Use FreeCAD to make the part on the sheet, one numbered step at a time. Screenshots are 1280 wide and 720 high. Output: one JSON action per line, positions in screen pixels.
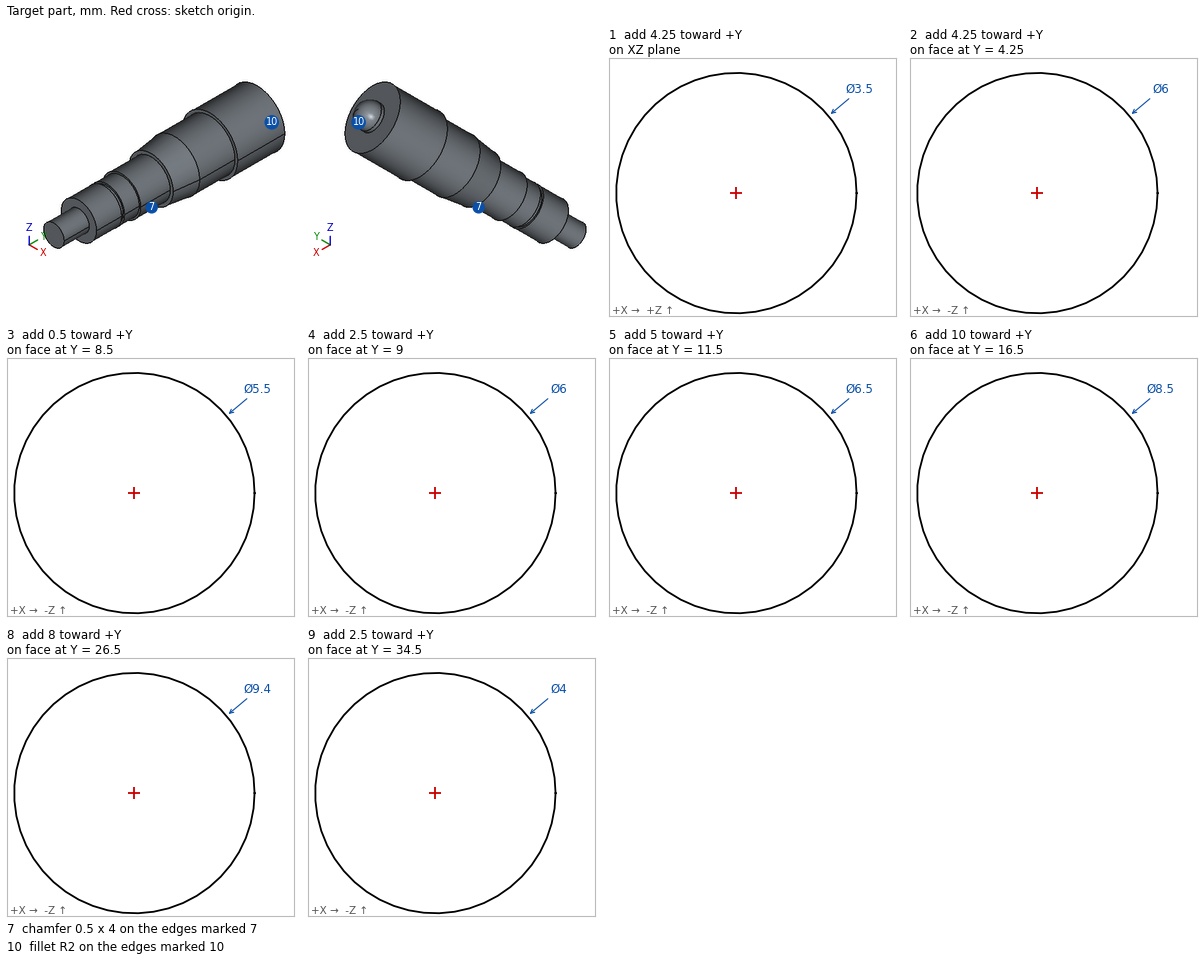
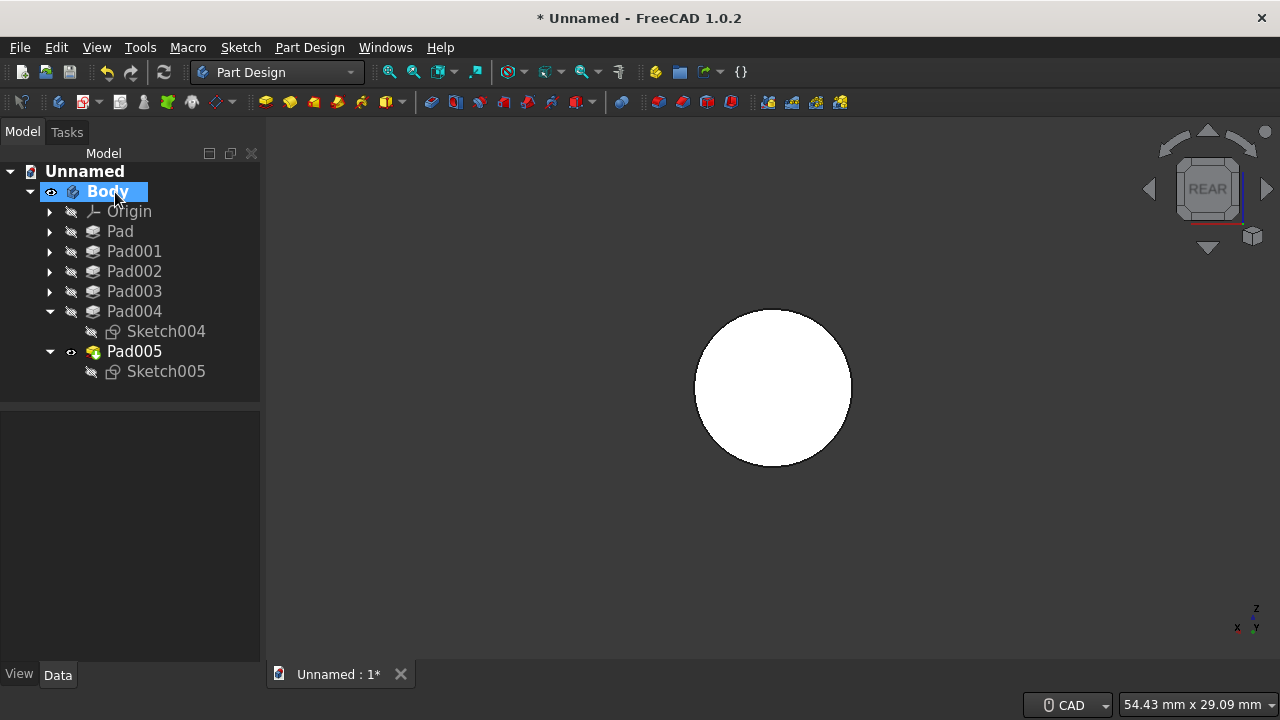
{"action": "key", "text": "0"}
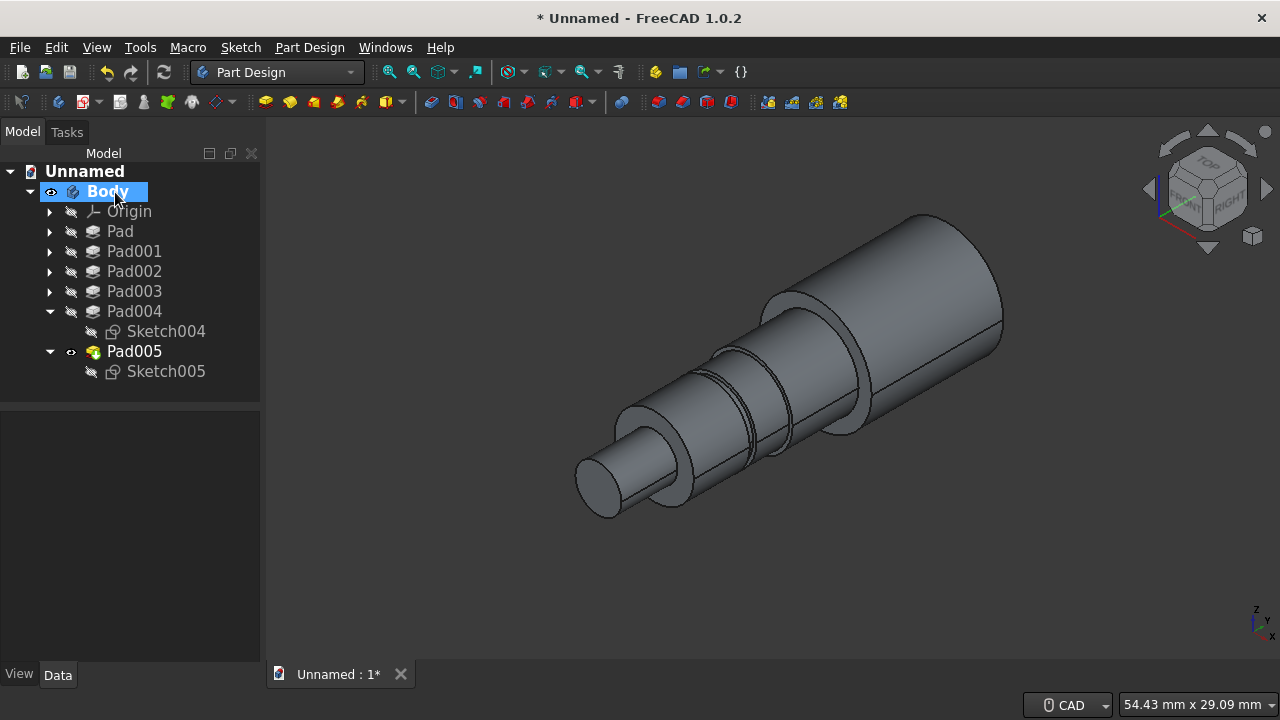
{"action": "left_click", "coordinate": [798, 291]}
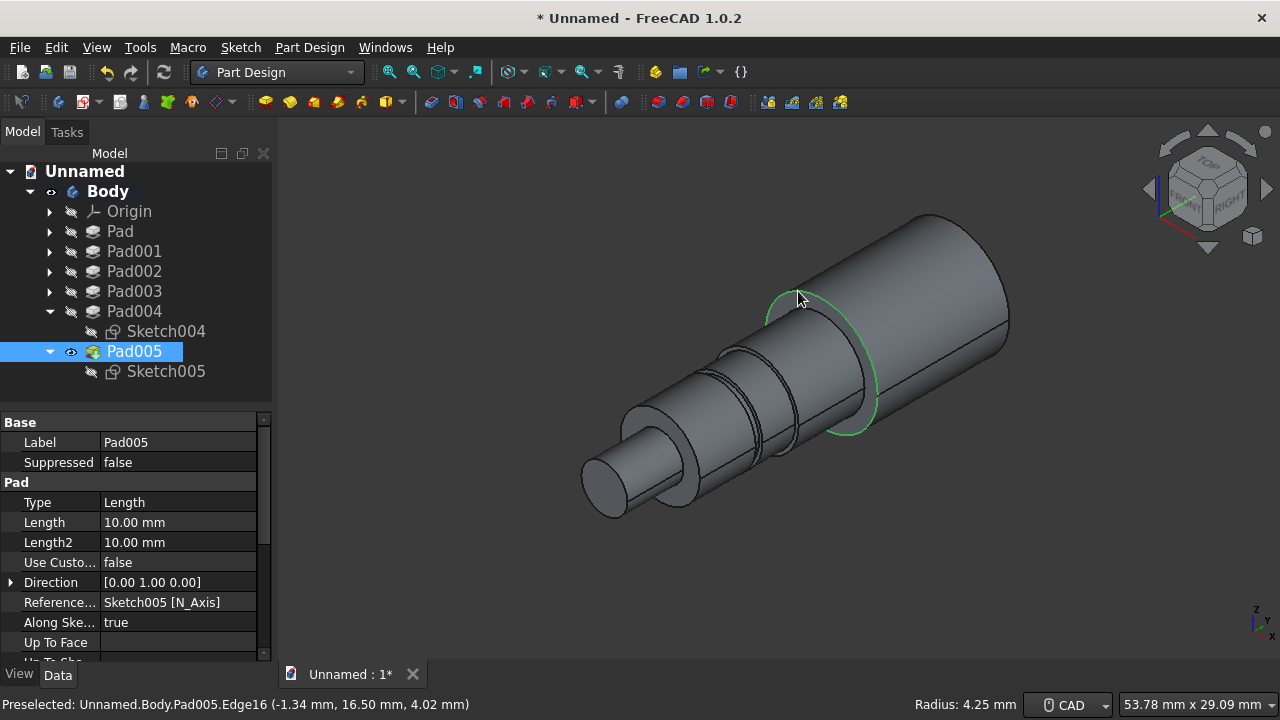
{"action": "left_click", "coordinate": [684, 102]}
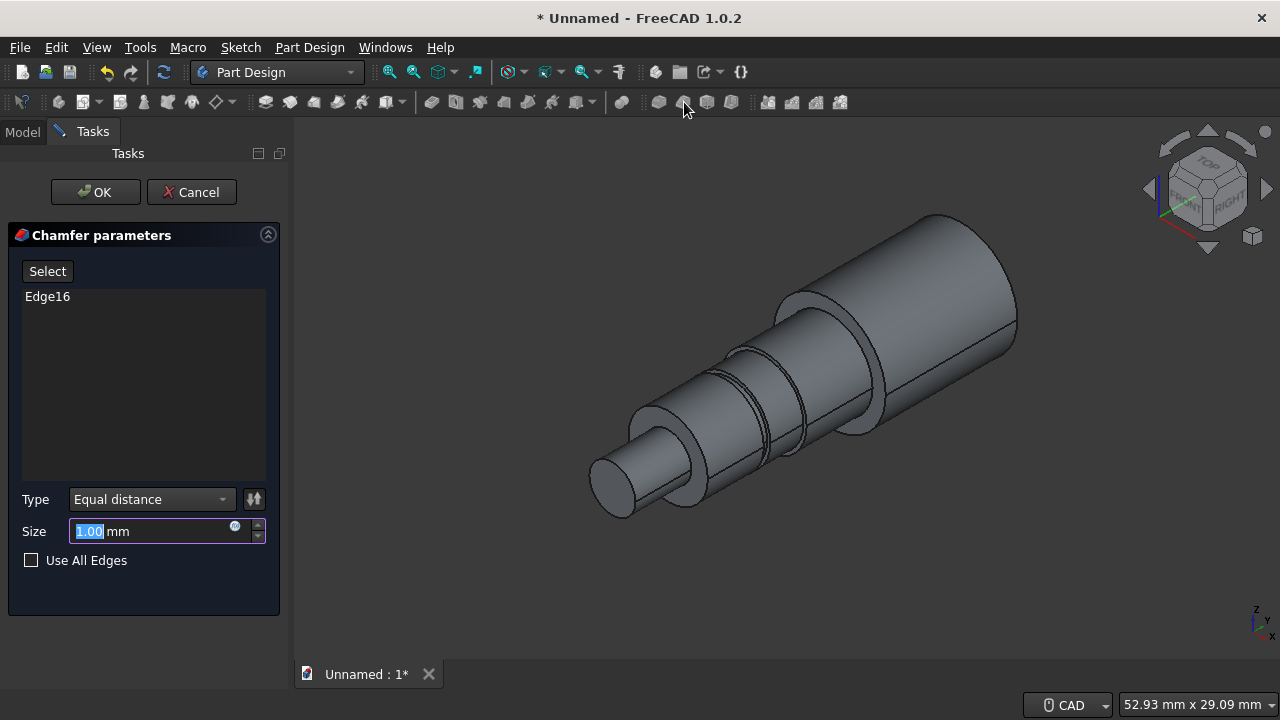
{"action": "type", "text": "0.5"}
{"action": "key", "text": "Tab"}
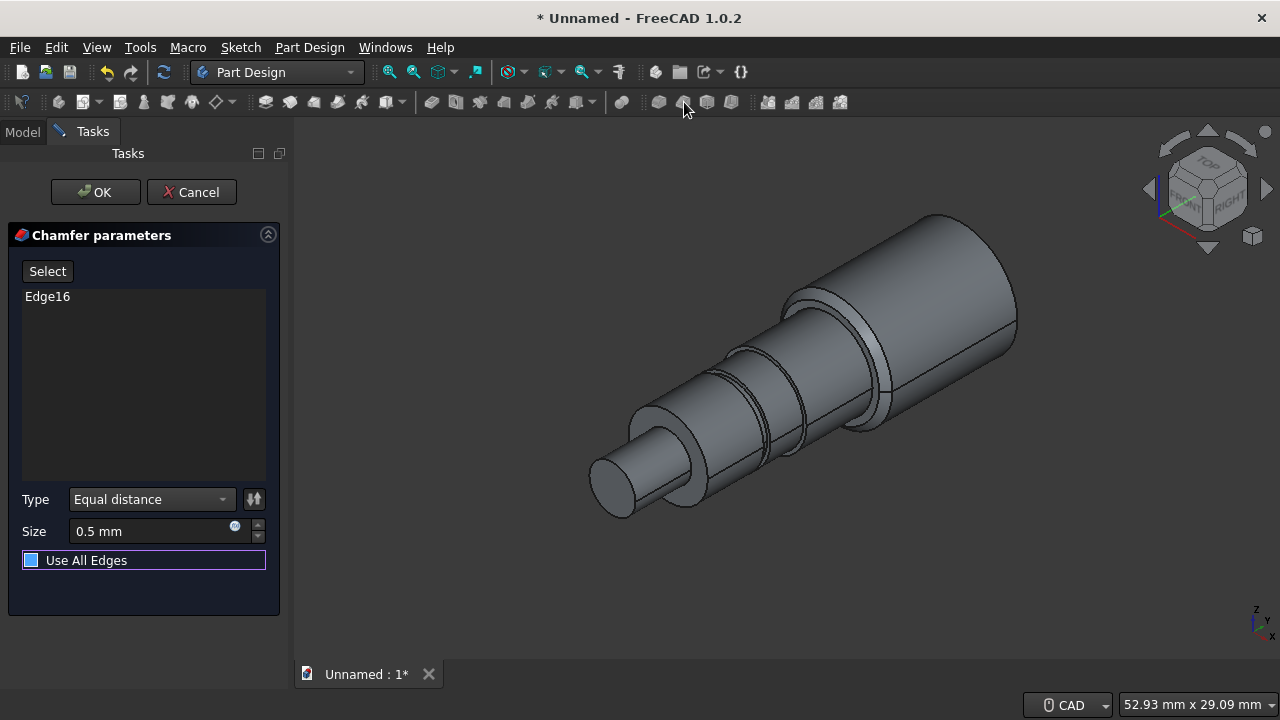
{"action": "left_click", "coordinate": [153, 500]}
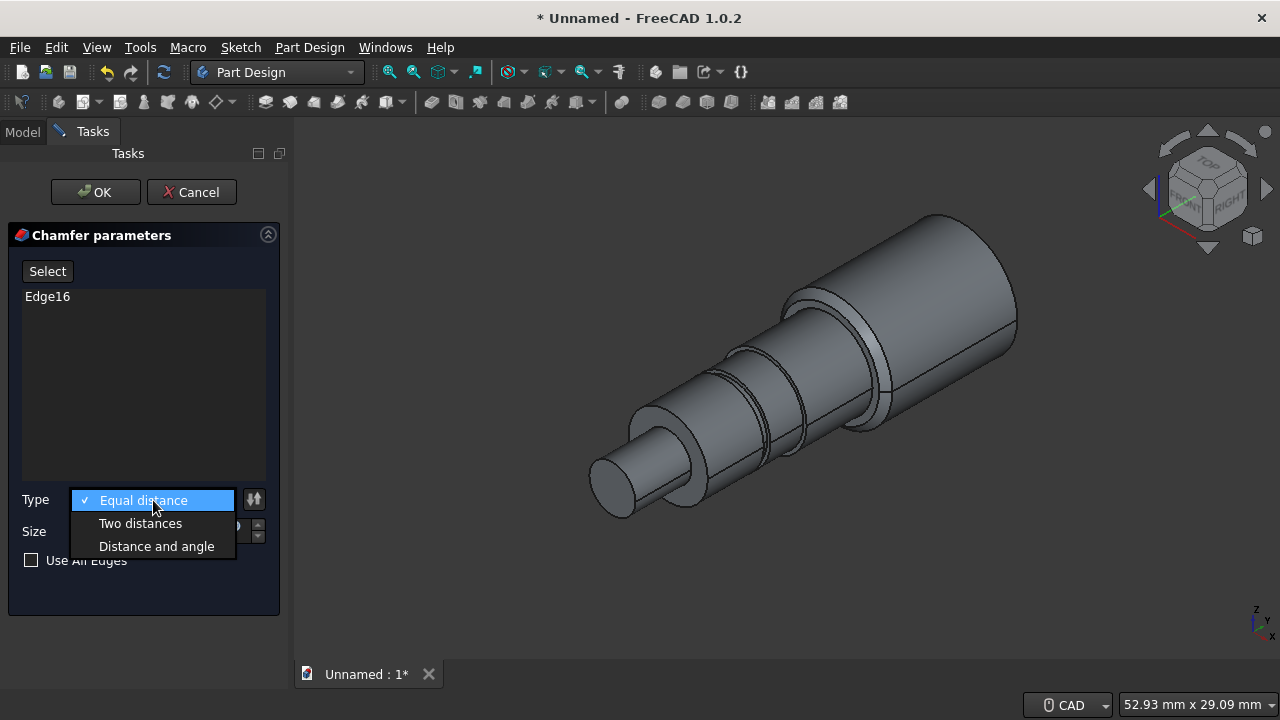
{"action": "left_click", "coordinate": [152, 524]}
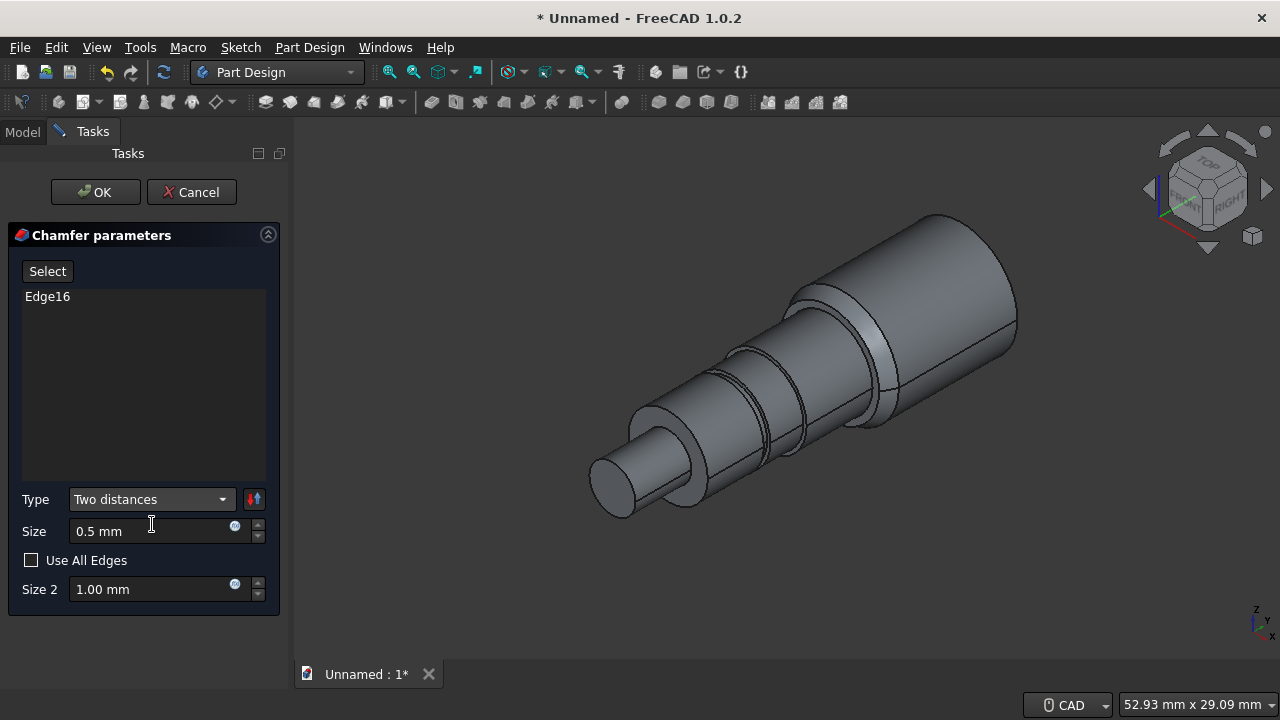
{"action": "triple_click", "coordinate": [160, 589]}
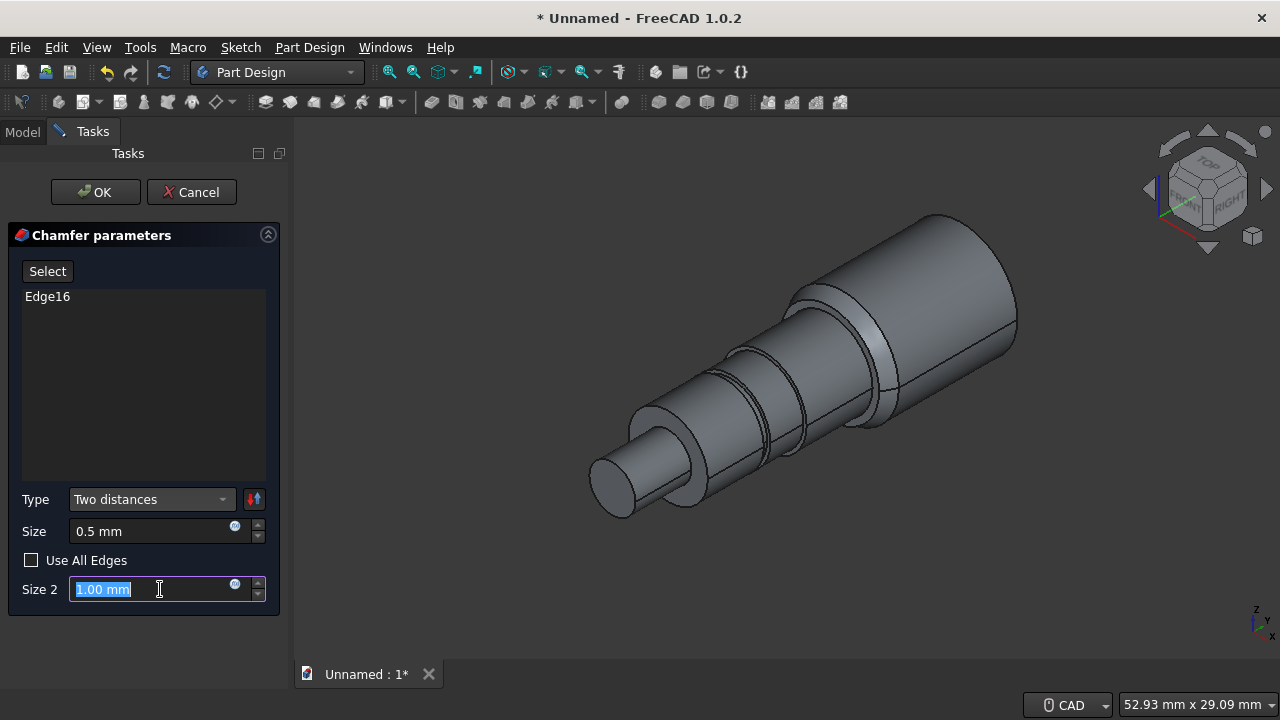
{"action": "type", "text": "4"}
{"action": "key", "text": "Tab"}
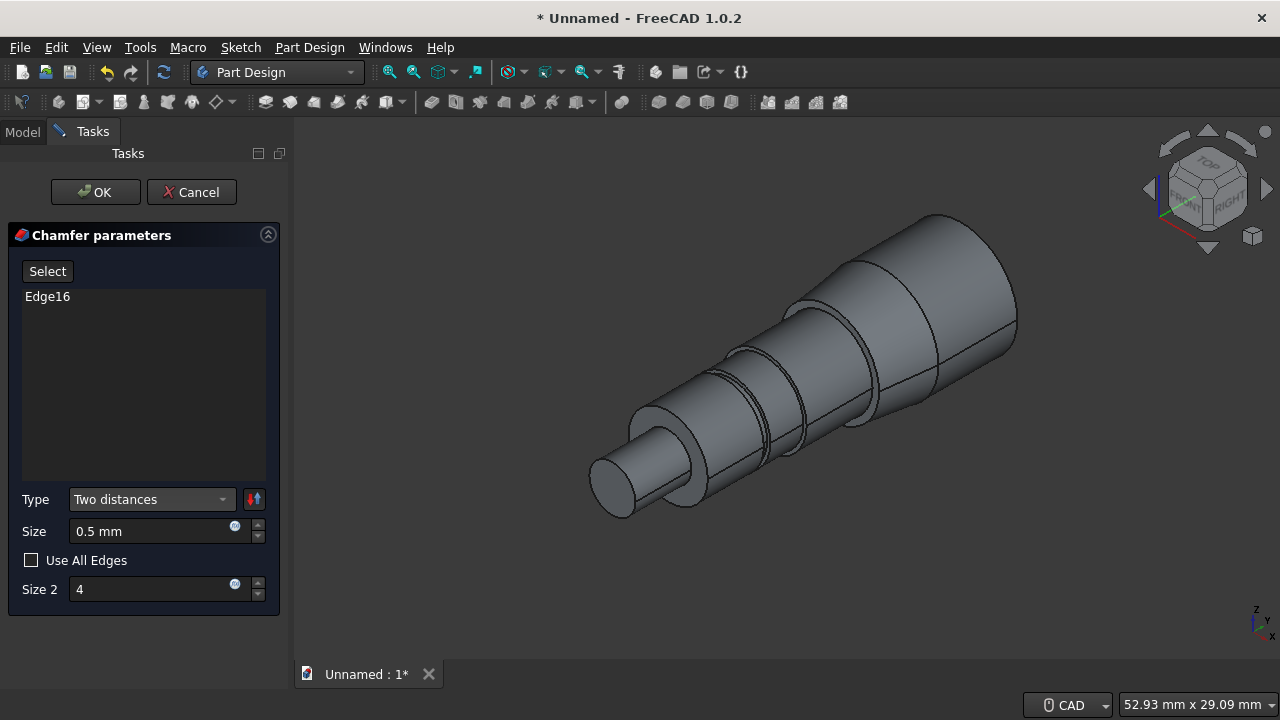
{"action": "left_click", "coordinate": [96, 192]}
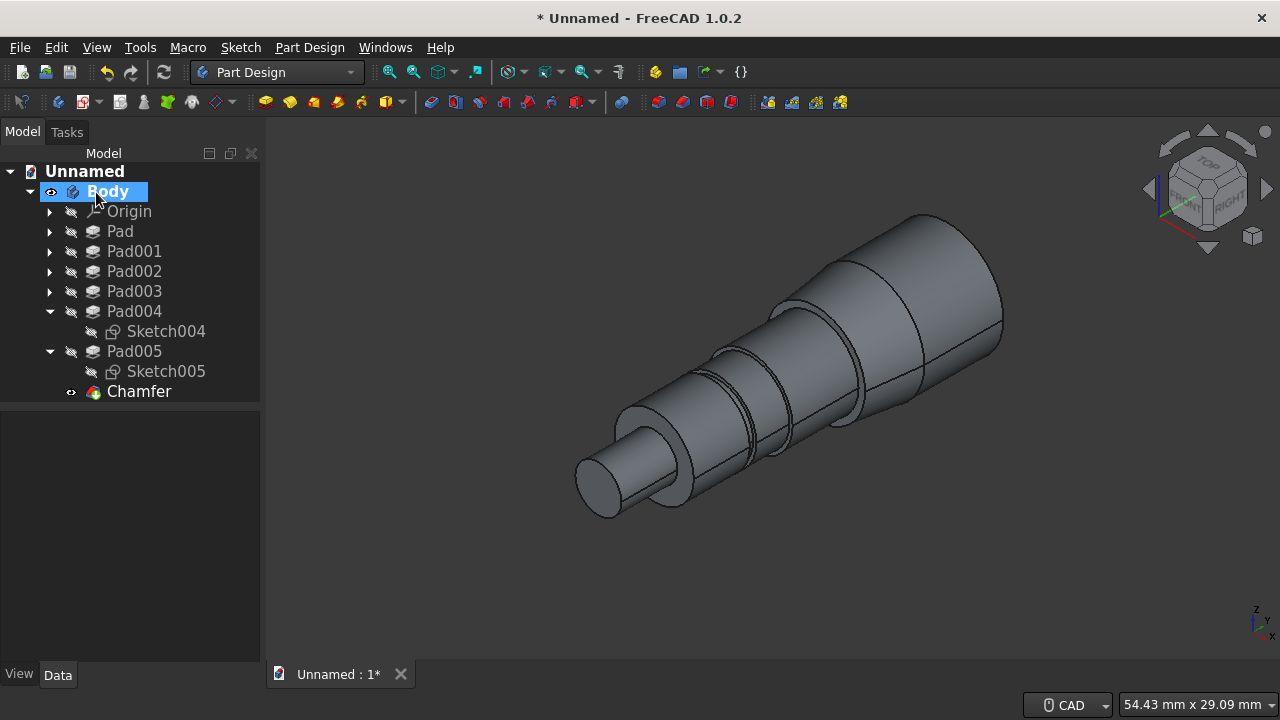
{"action": "key", "text": "4"}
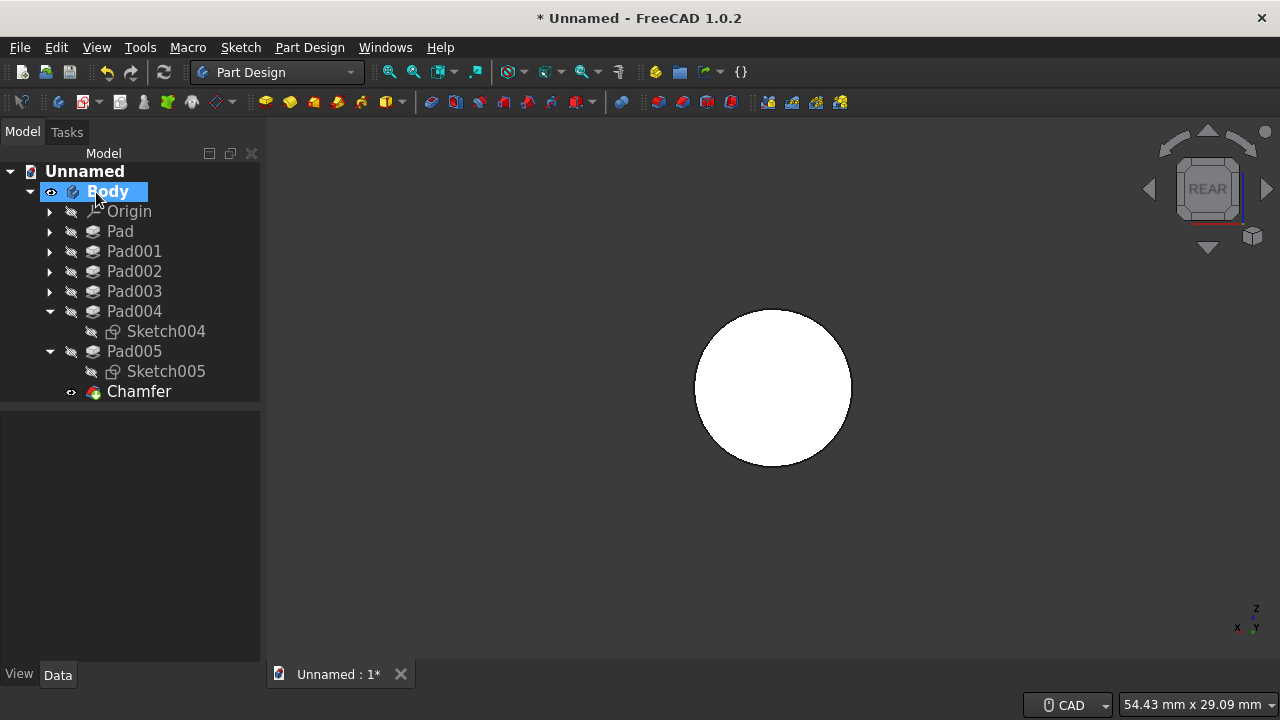
{"action": "left_click", "coordinate": [390, 72]}